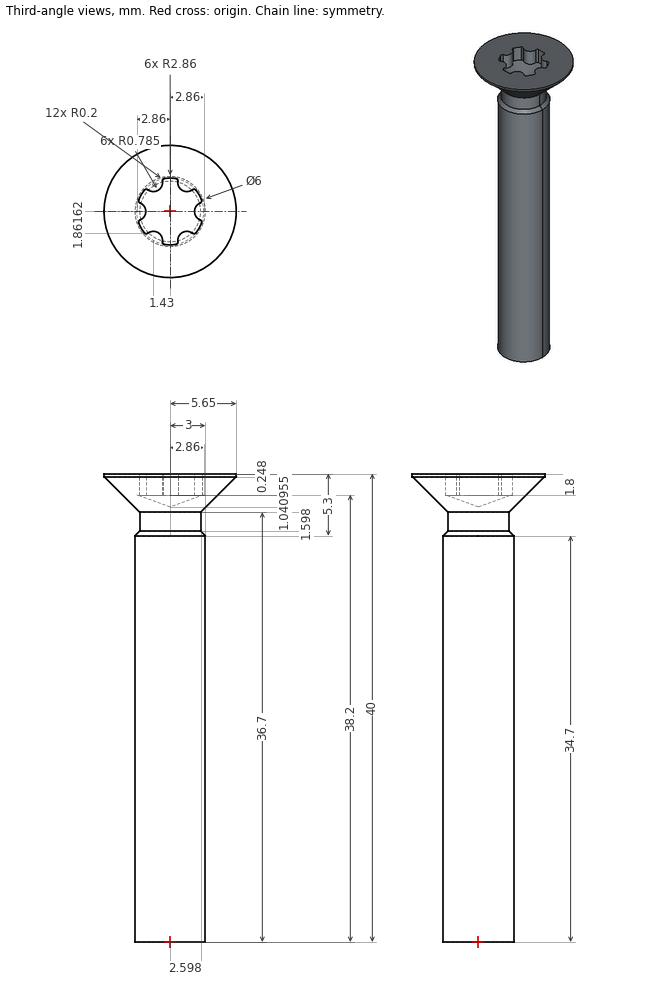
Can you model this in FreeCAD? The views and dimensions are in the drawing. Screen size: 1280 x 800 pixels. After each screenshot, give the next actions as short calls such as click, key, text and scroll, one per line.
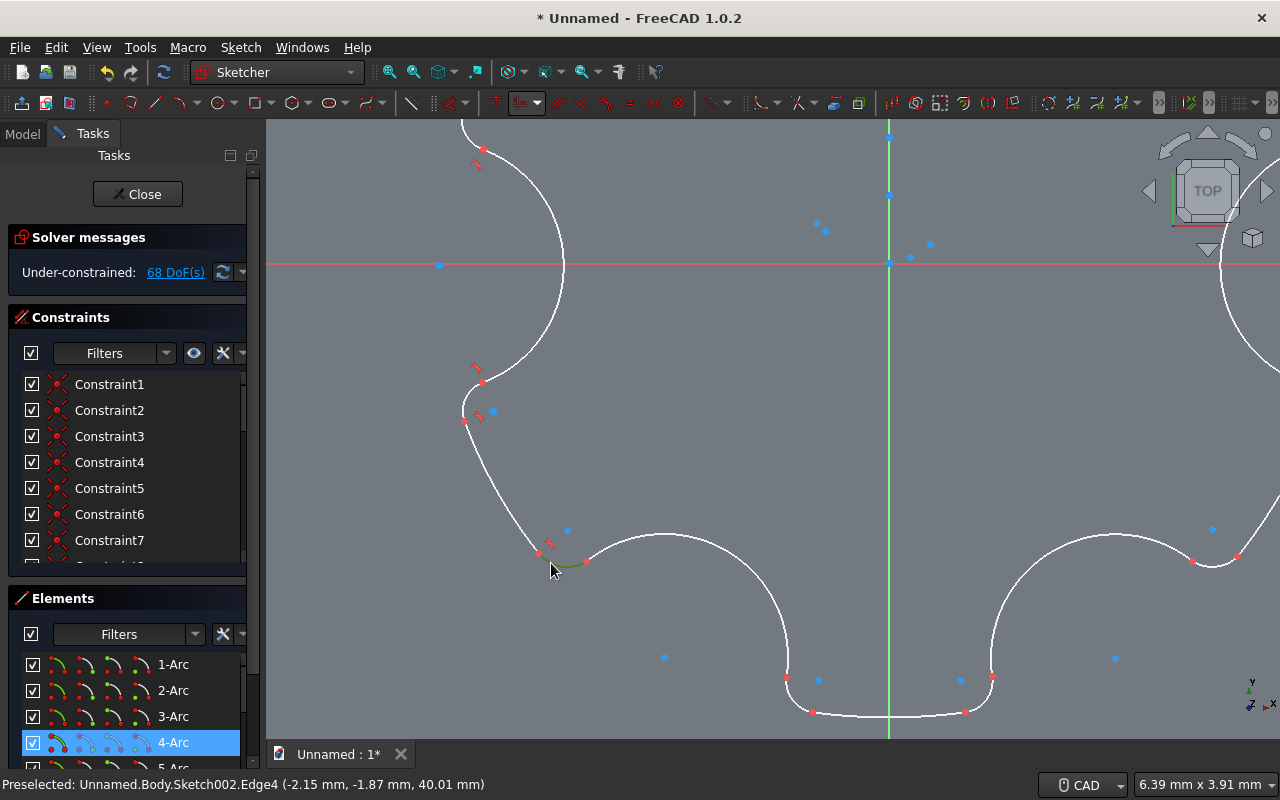
click(769, 592)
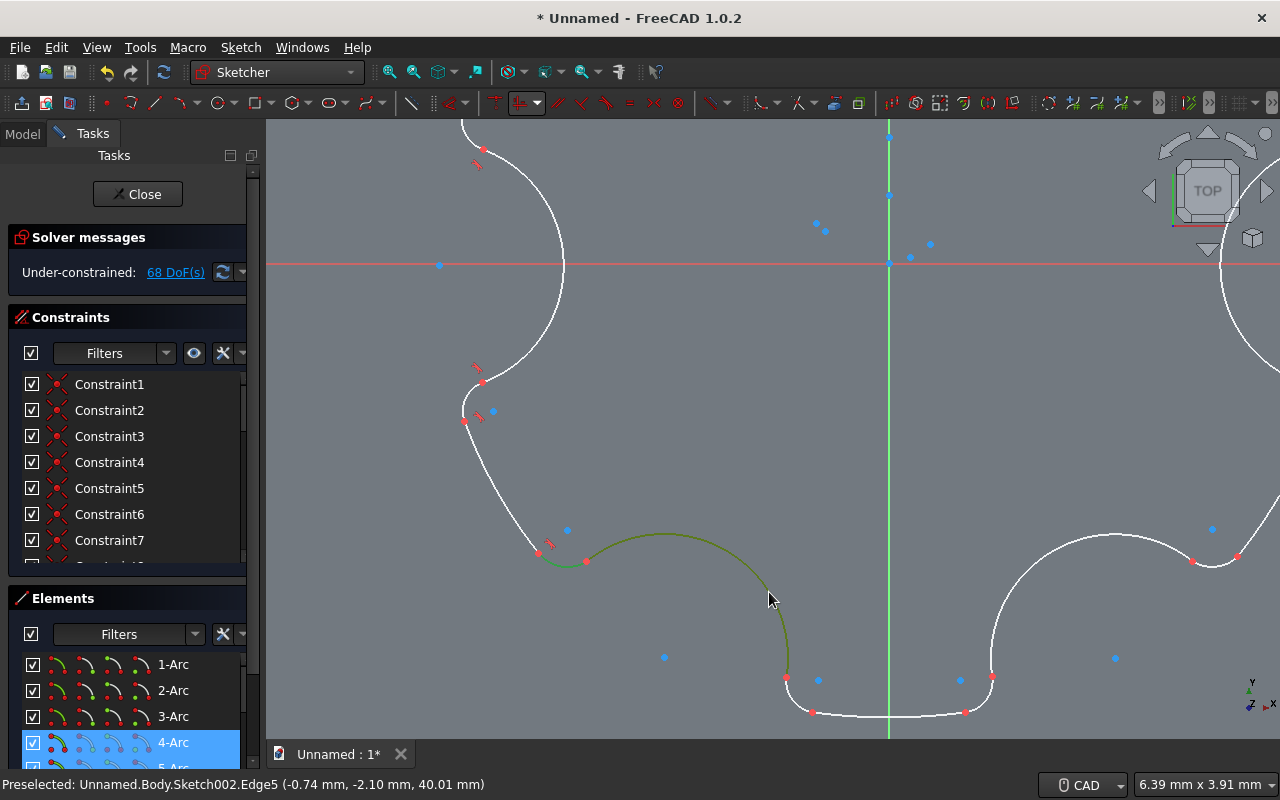
click(606, 104)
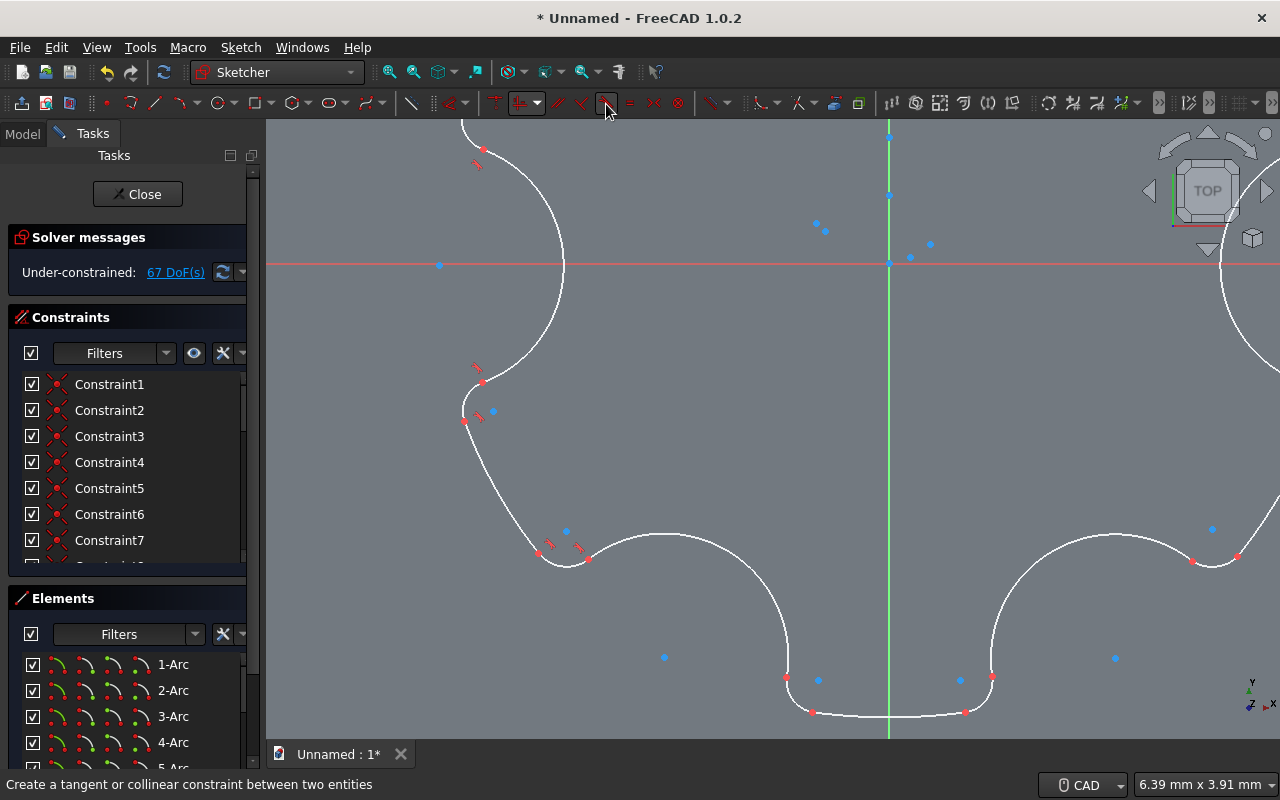
click(770, 592)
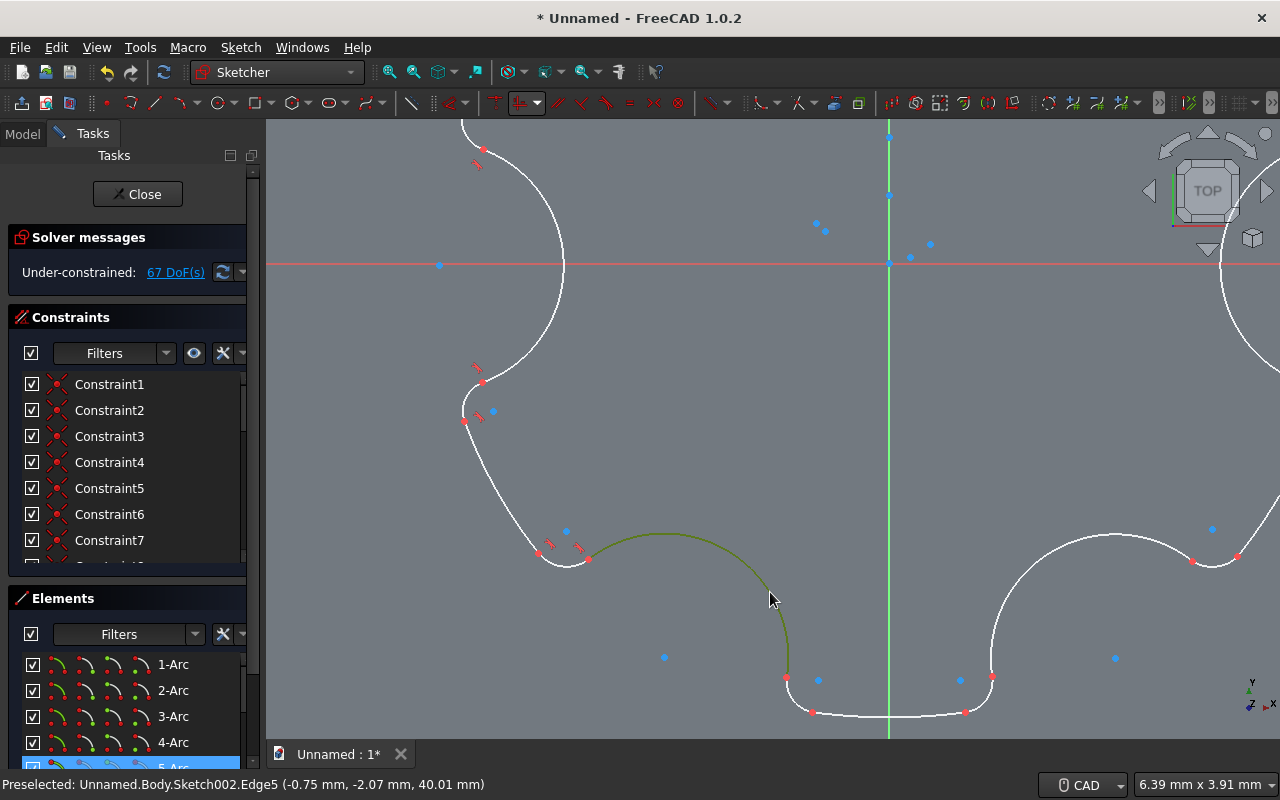
click(789, 692)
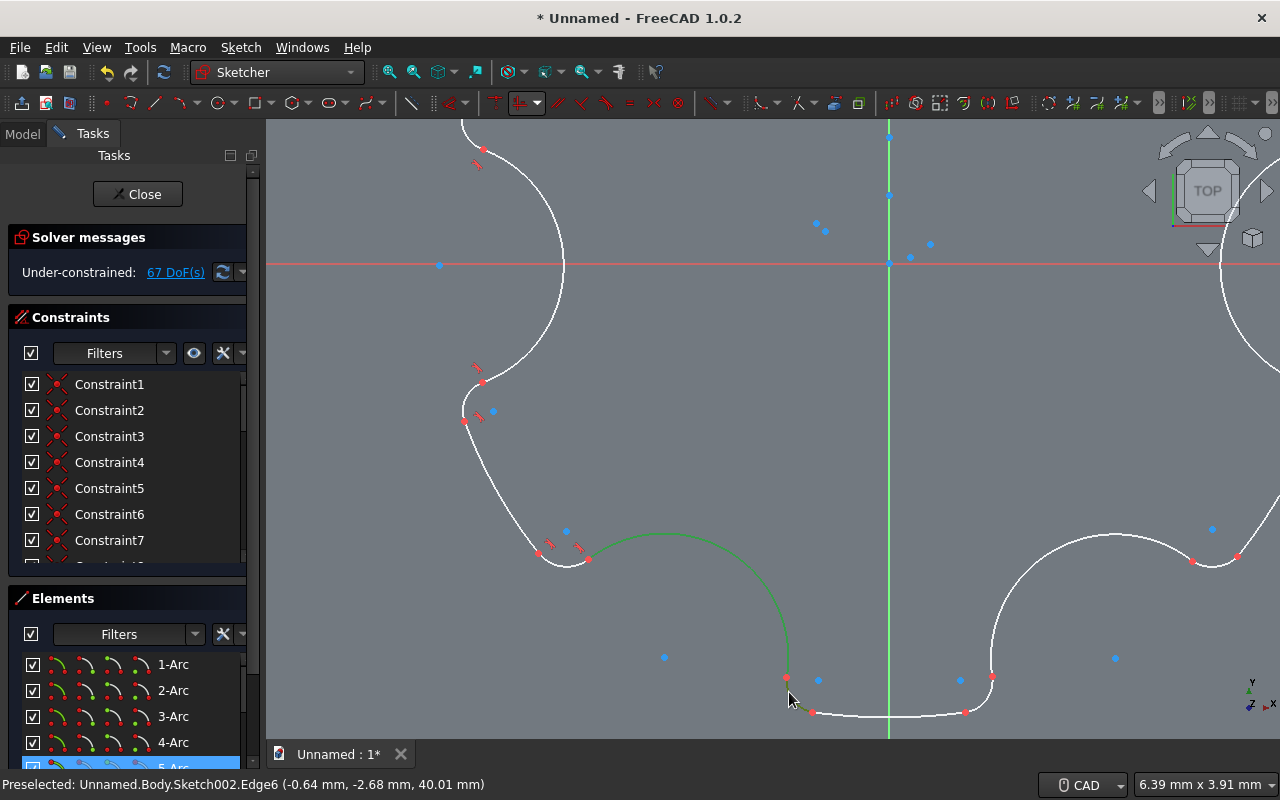
click(606, 104)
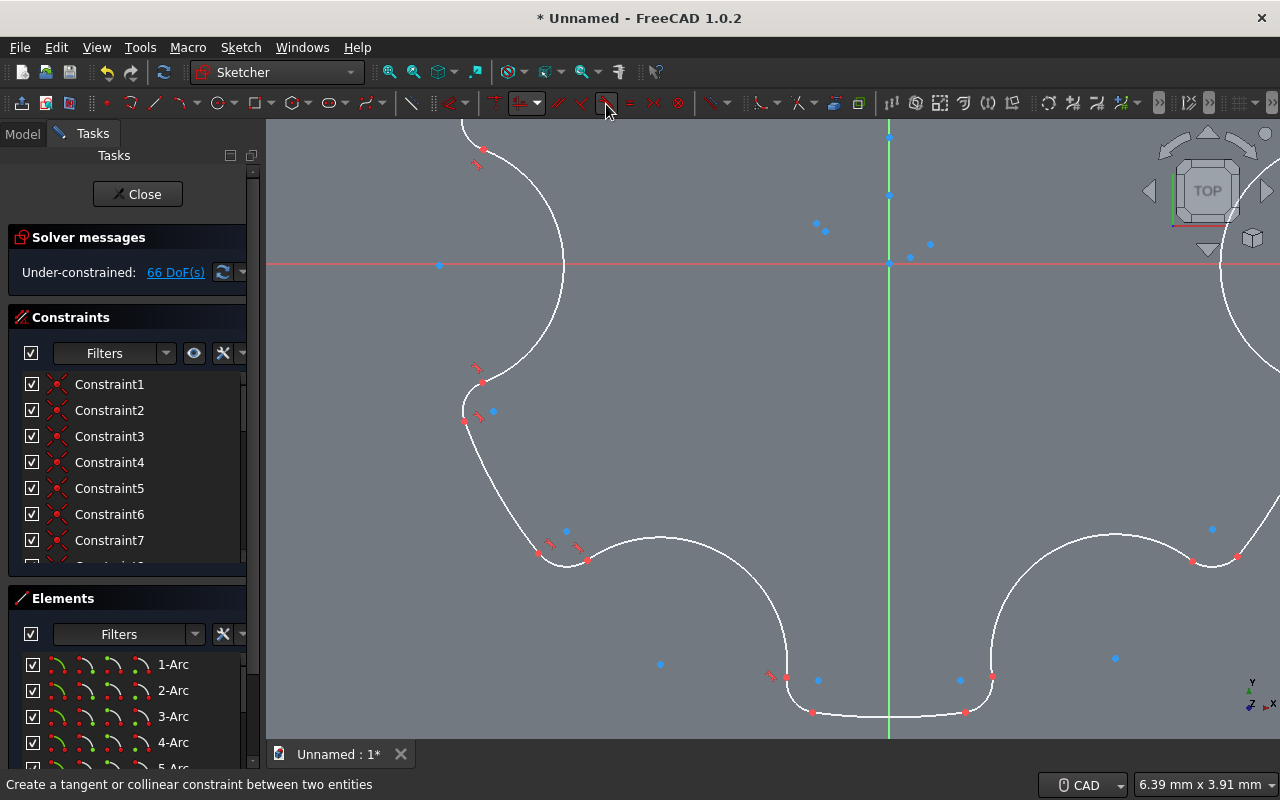
click(789, 692)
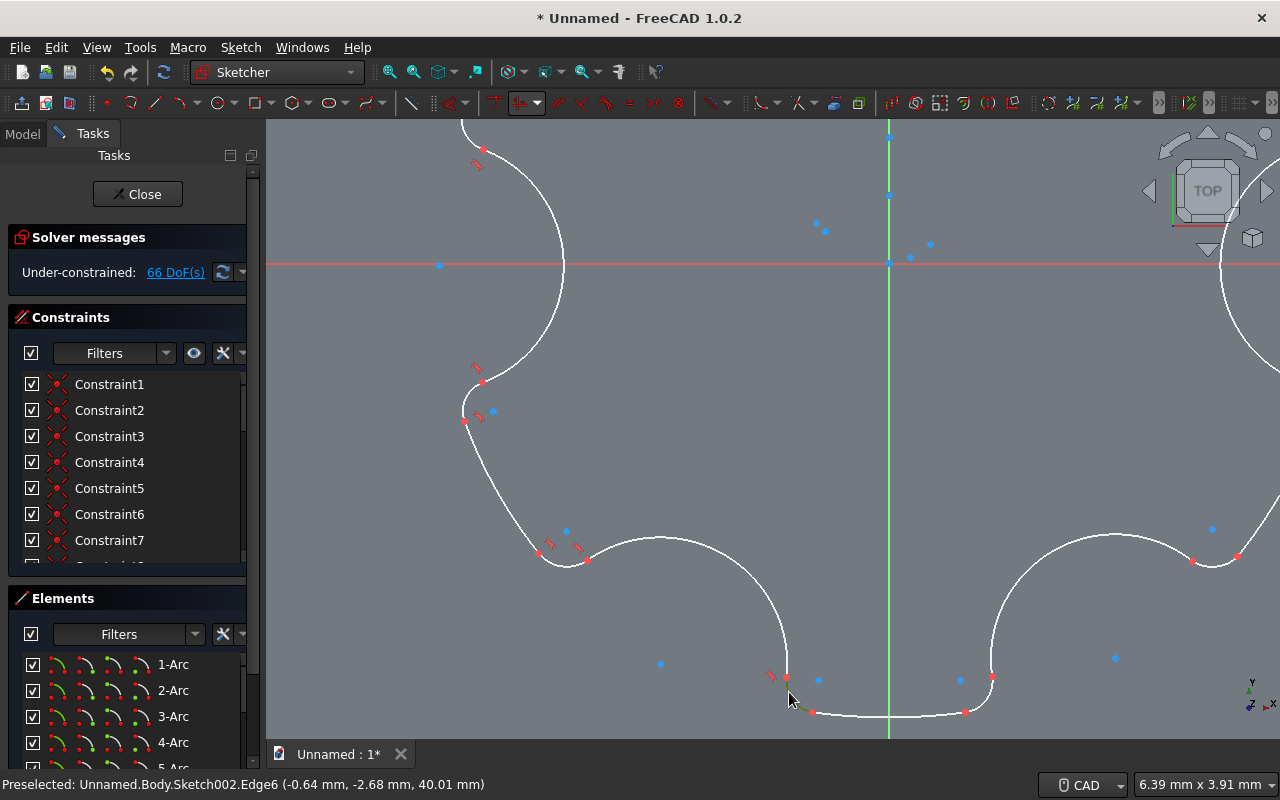
scroll(554, 564, down, 4)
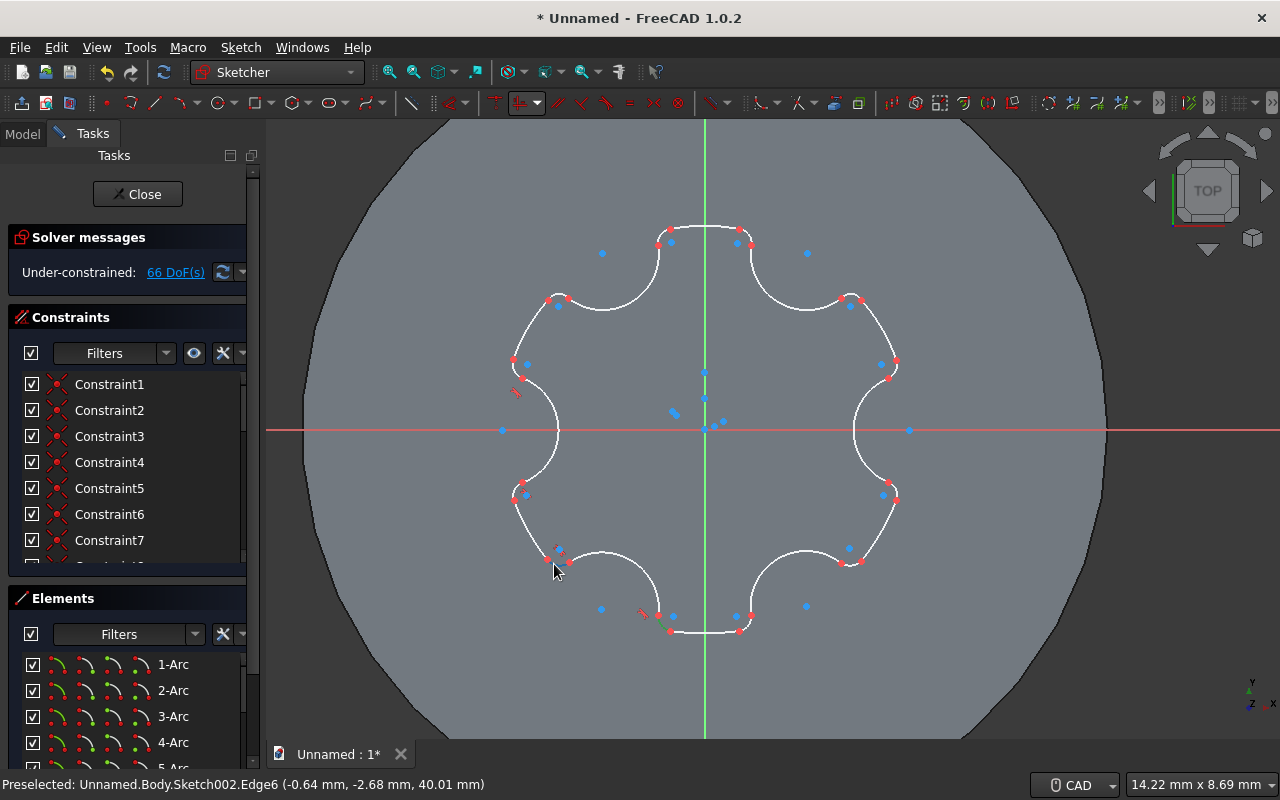
click(691, 633)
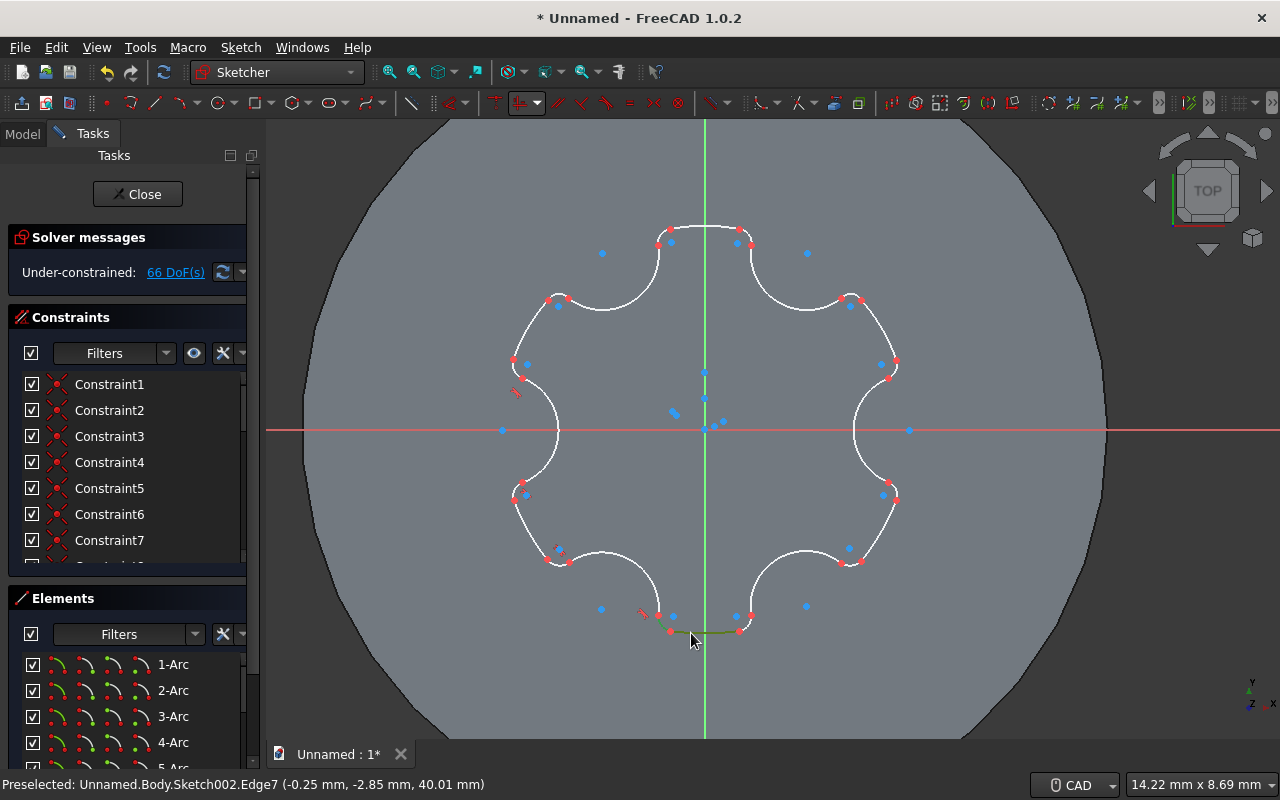
click(606, 104)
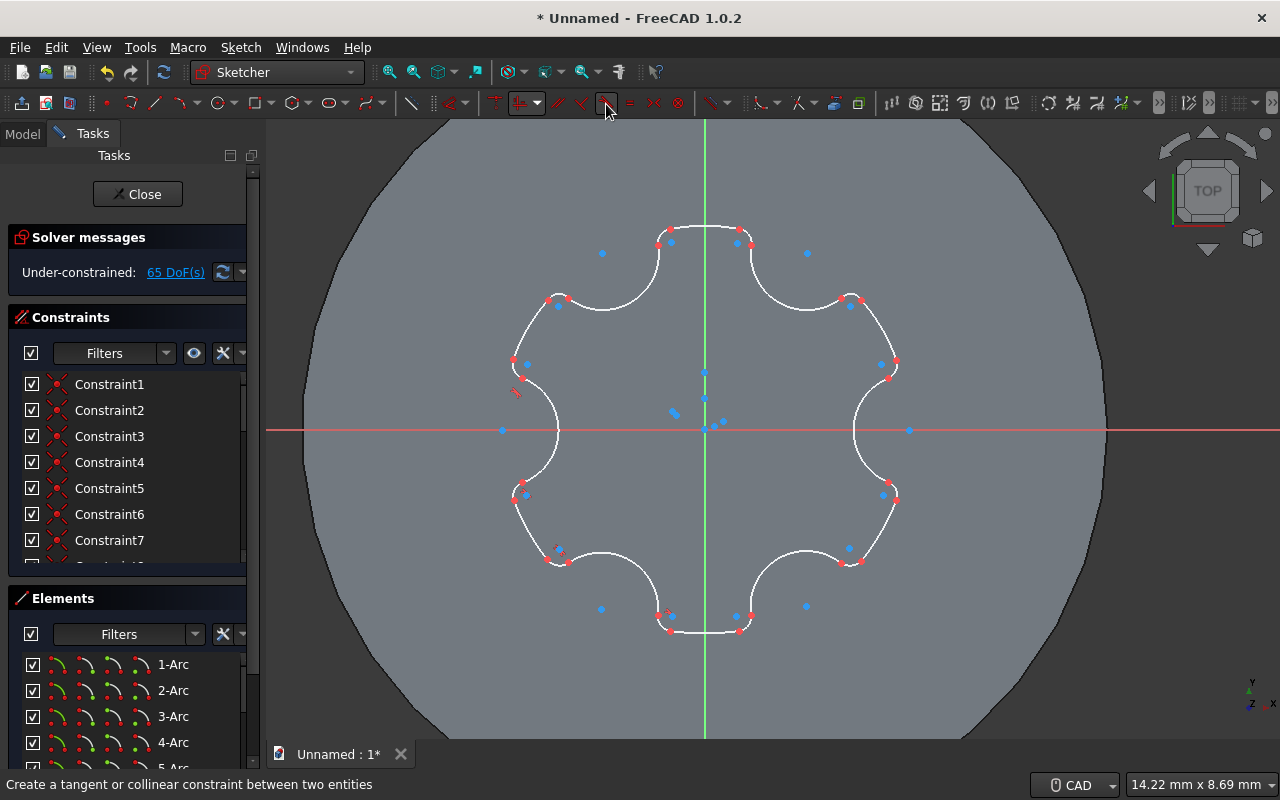
click(691, 633)